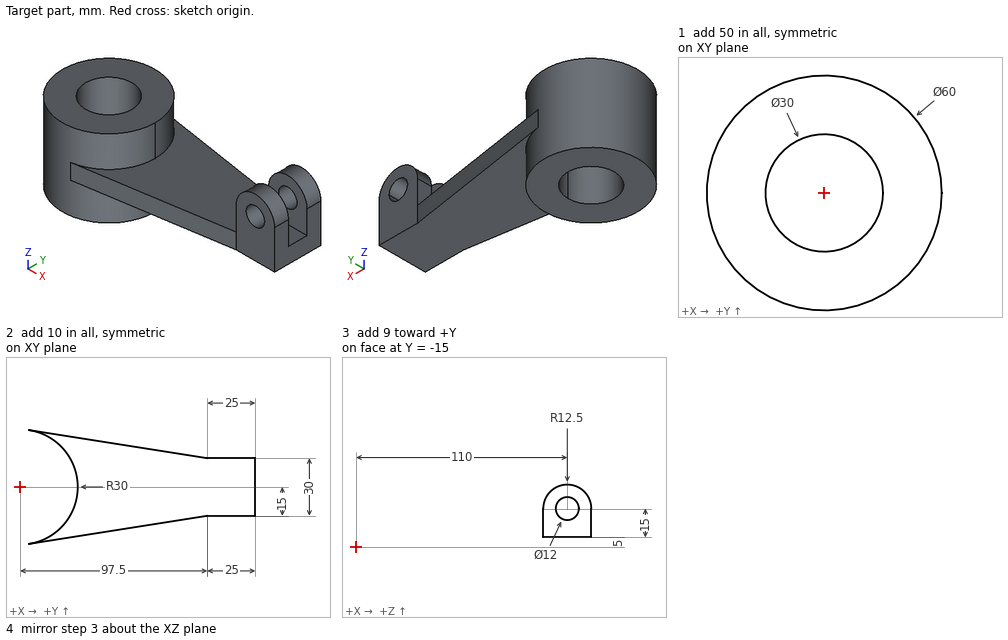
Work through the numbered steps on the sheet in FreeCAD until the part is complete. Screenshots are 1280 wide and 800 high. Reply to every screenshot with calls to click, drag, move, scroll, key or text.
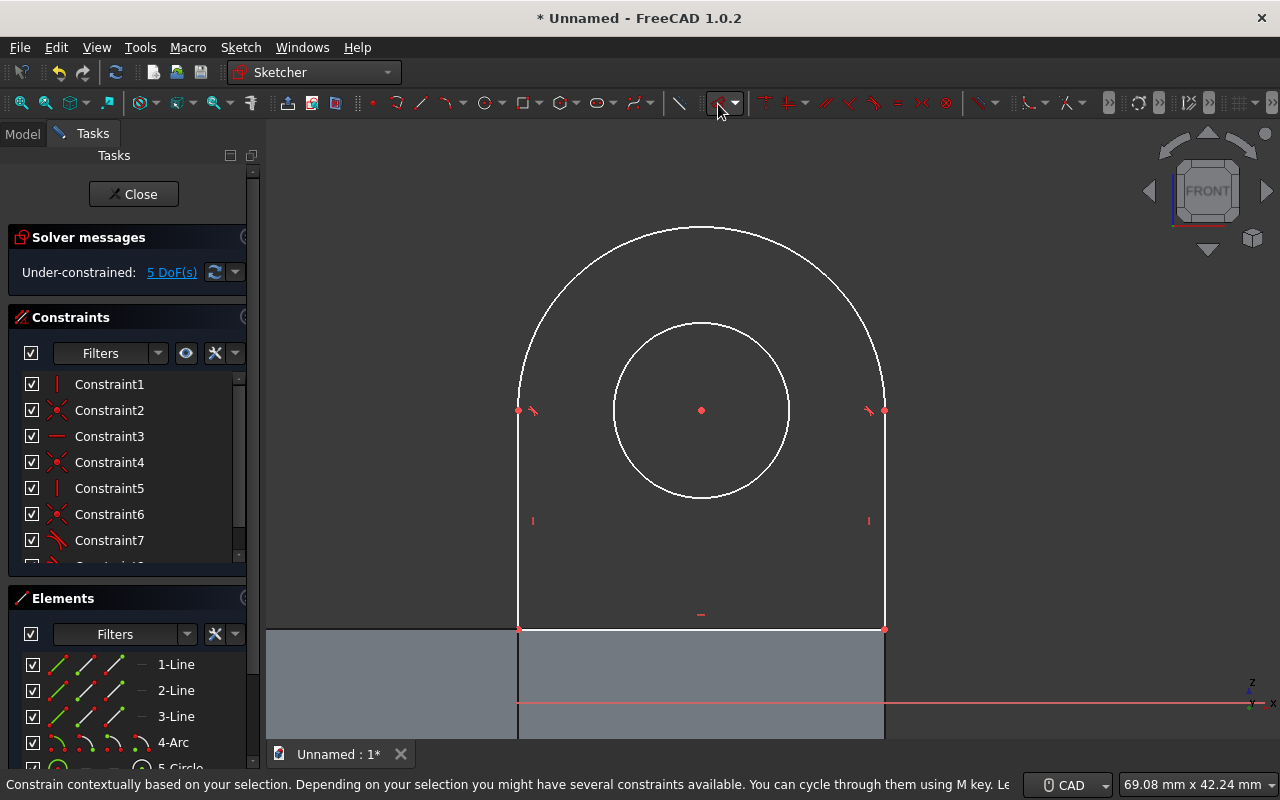
click(809, 262)
click(828, 236)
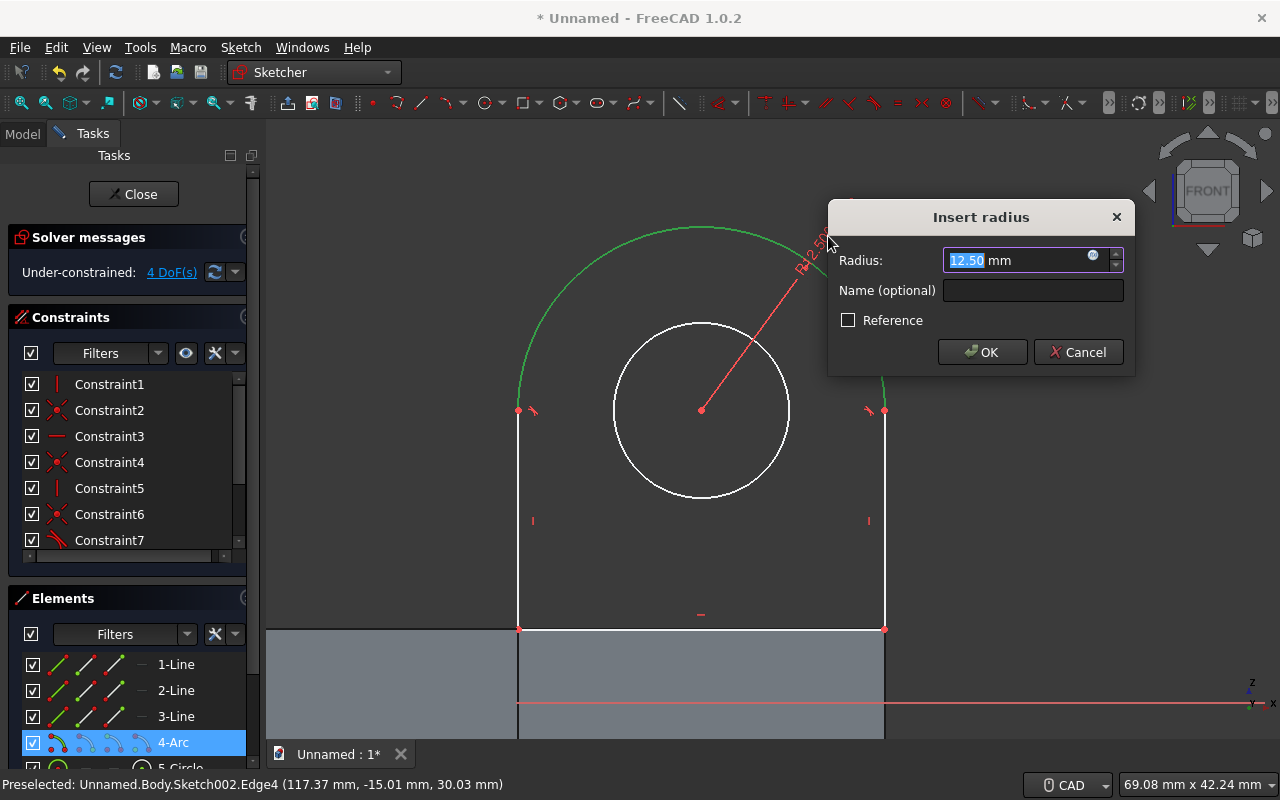
text(12.5)
key(Return)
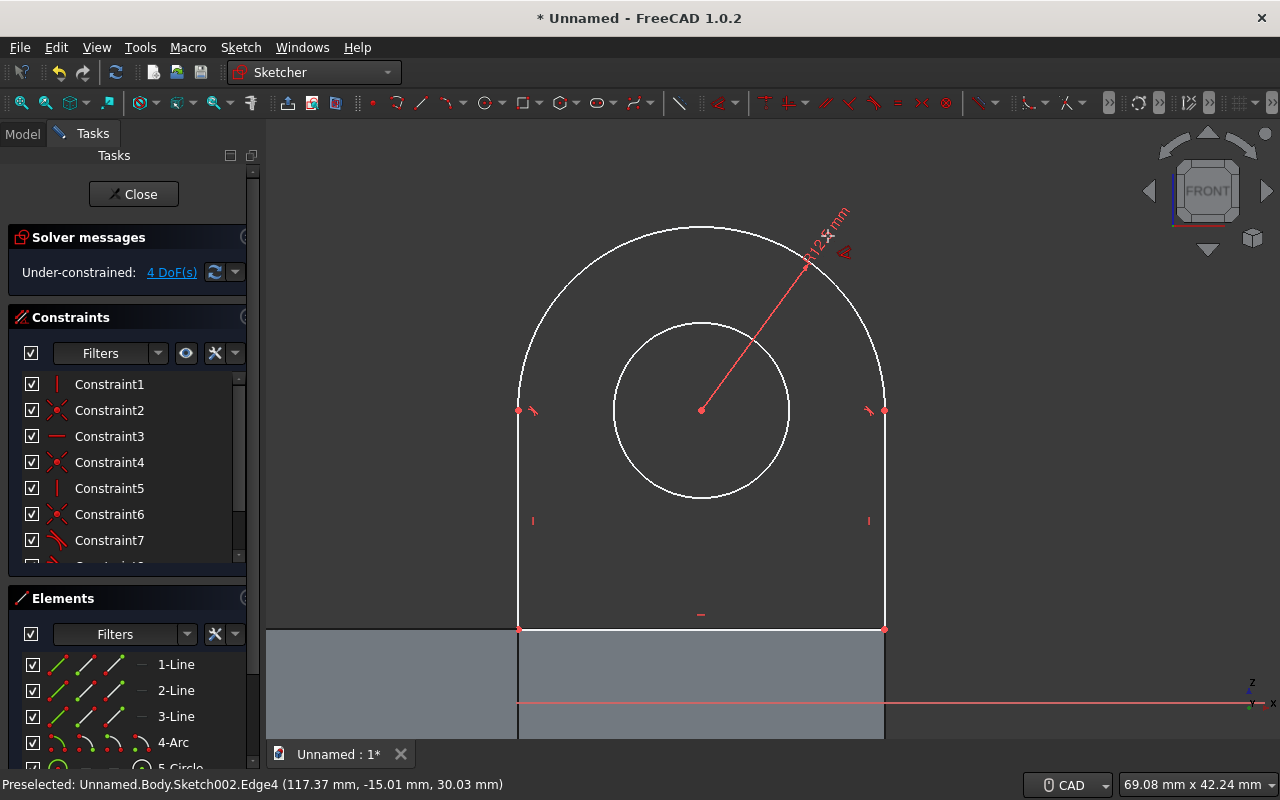
click(763, 348)
click(785, 325)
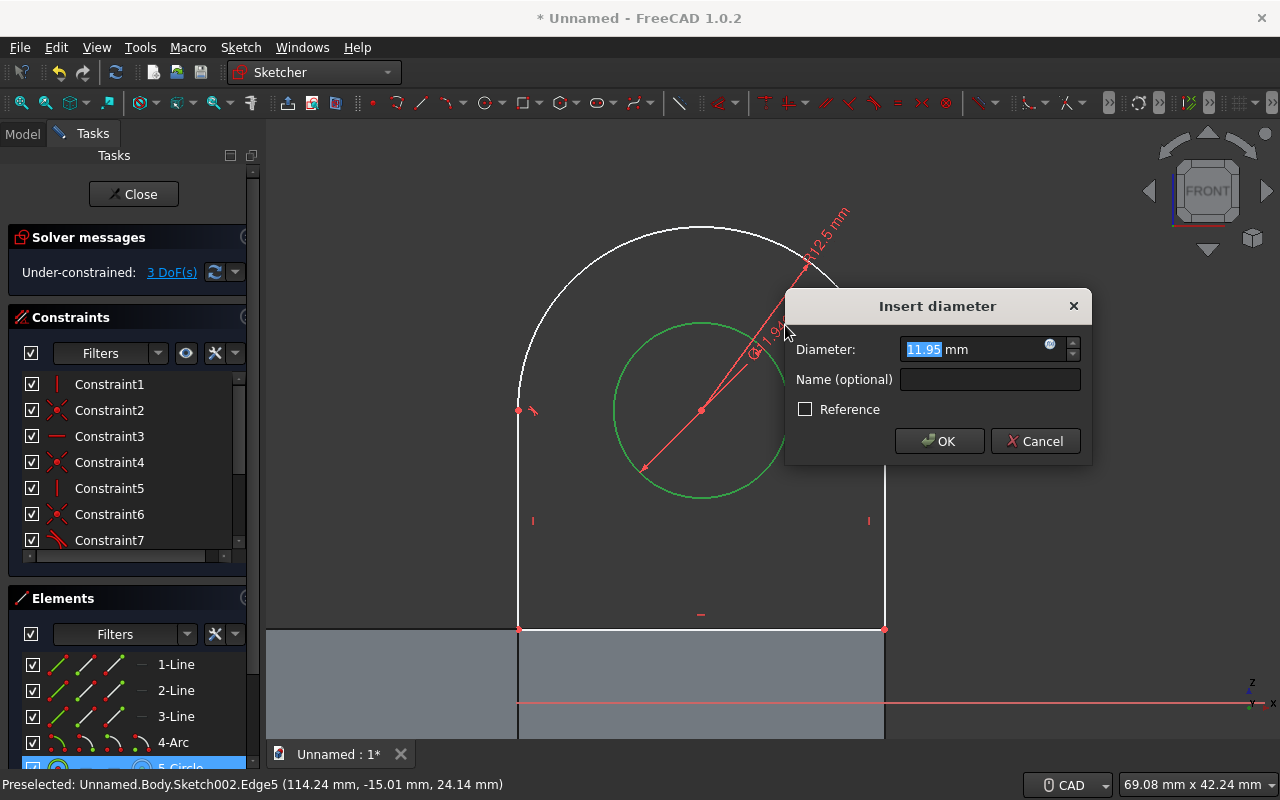
text(12)
key(Return)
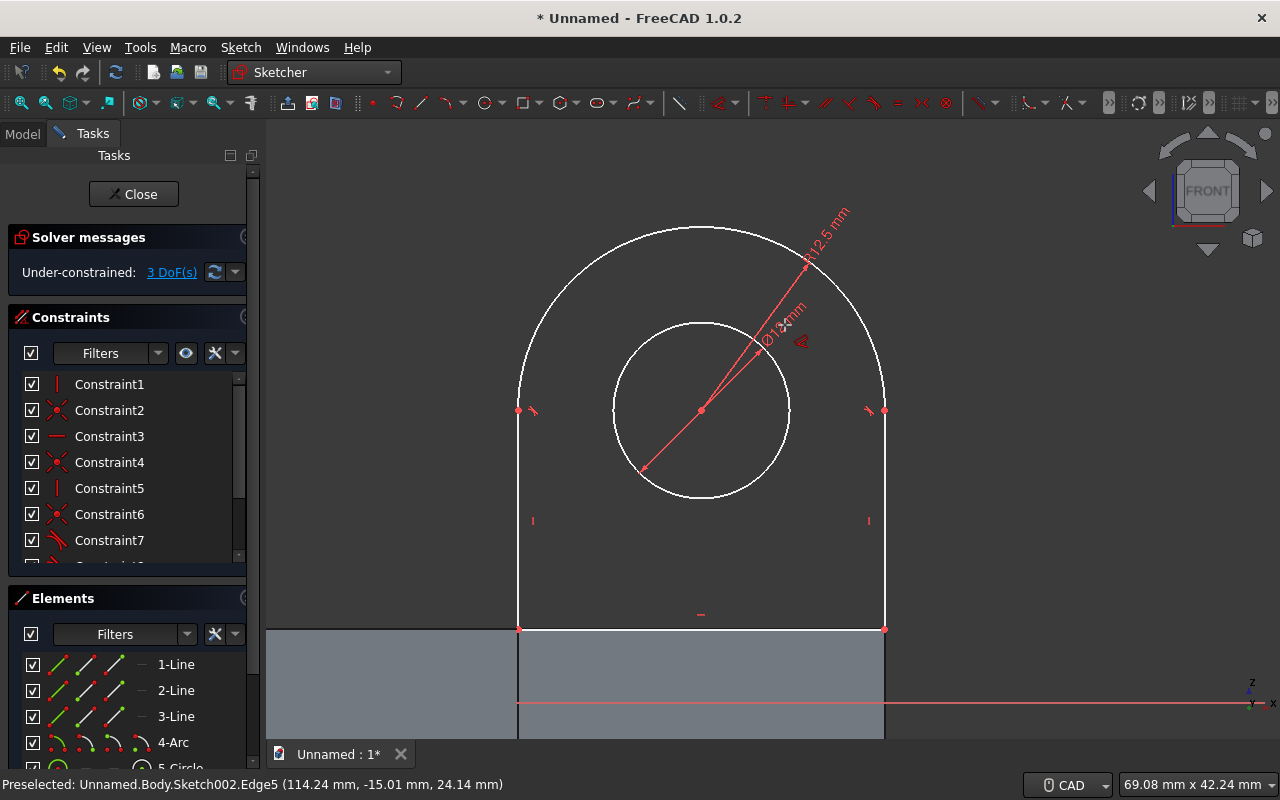
click(518, 476)
click(484, 520)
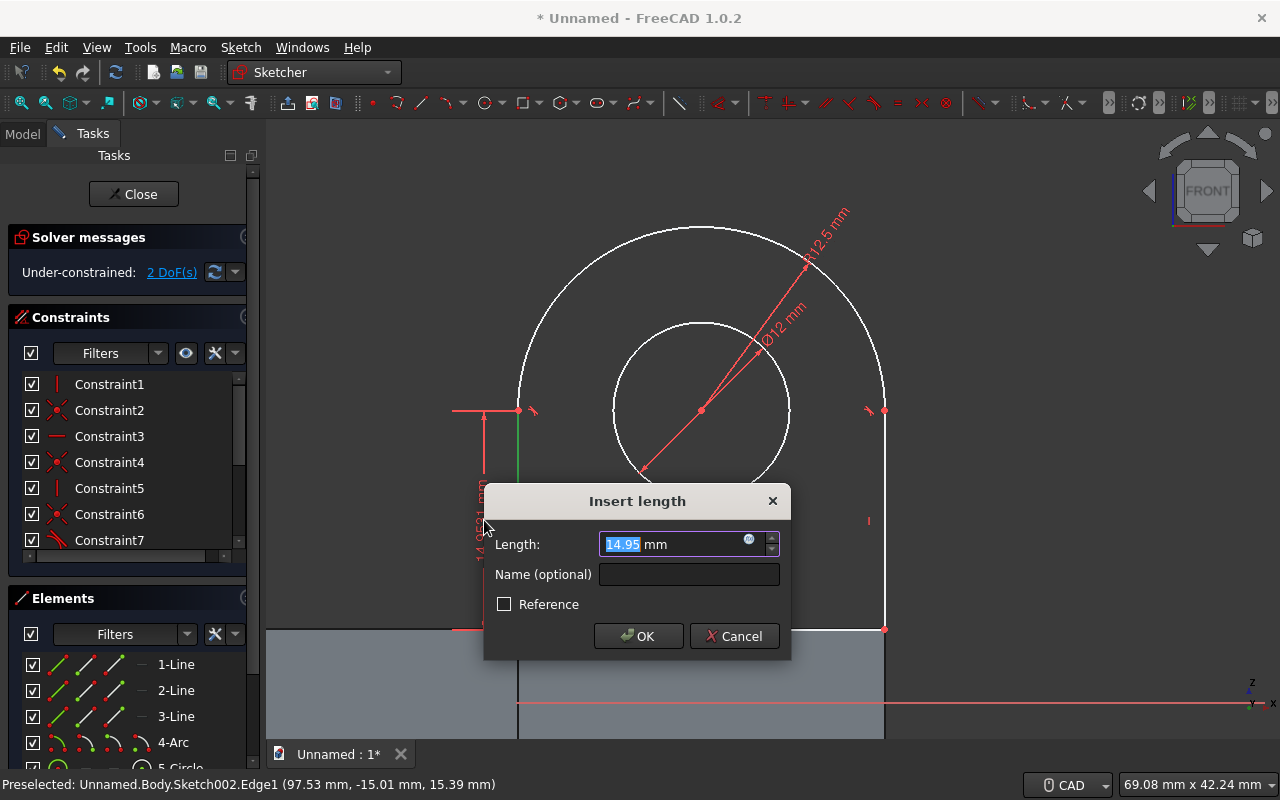
text(15)
key(Return)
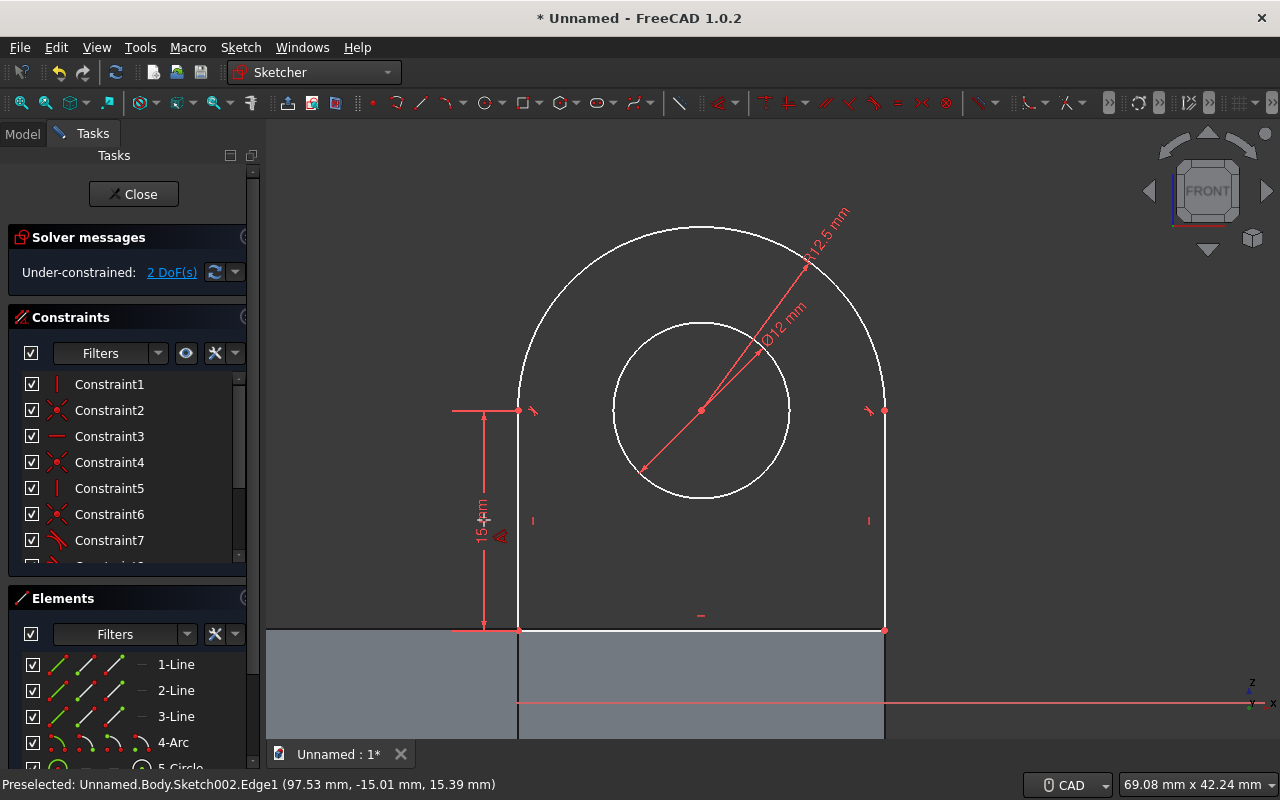
click(518, 631)
click(552, 667)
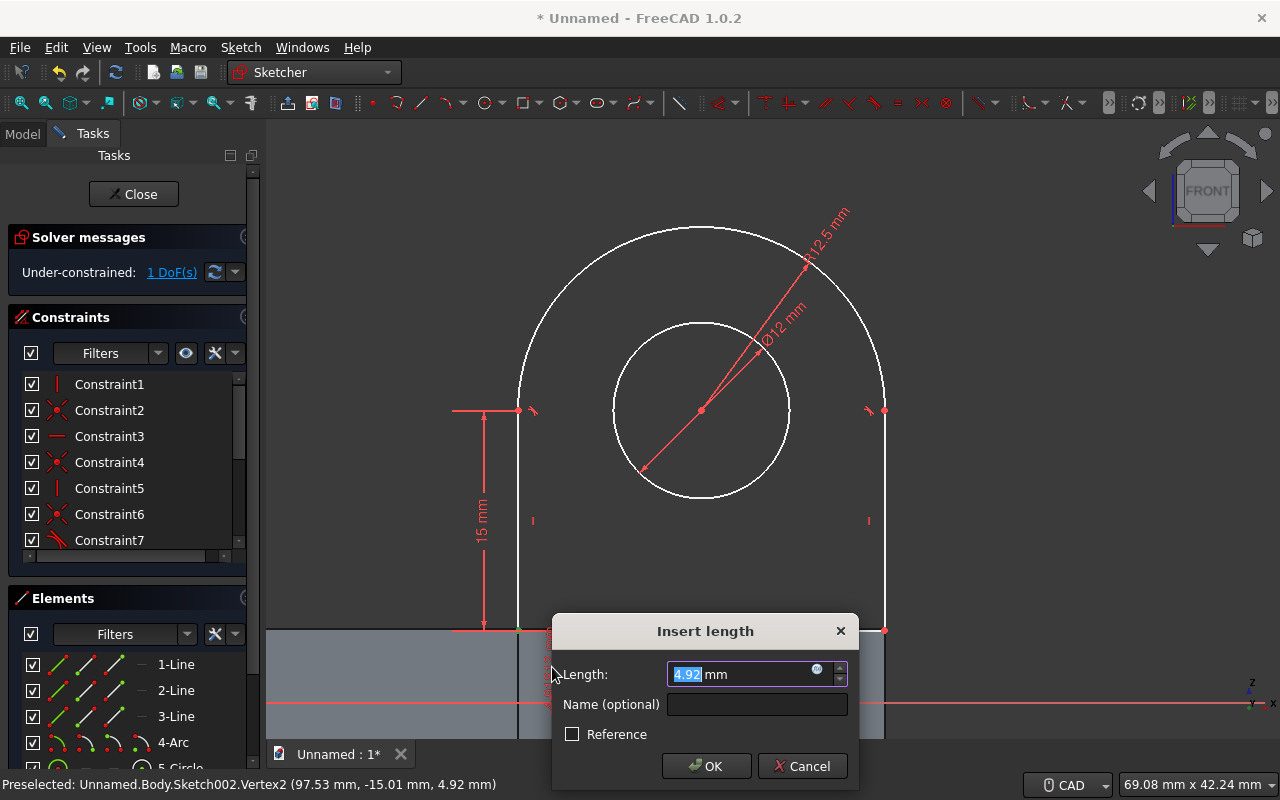
text(5)
key(Return)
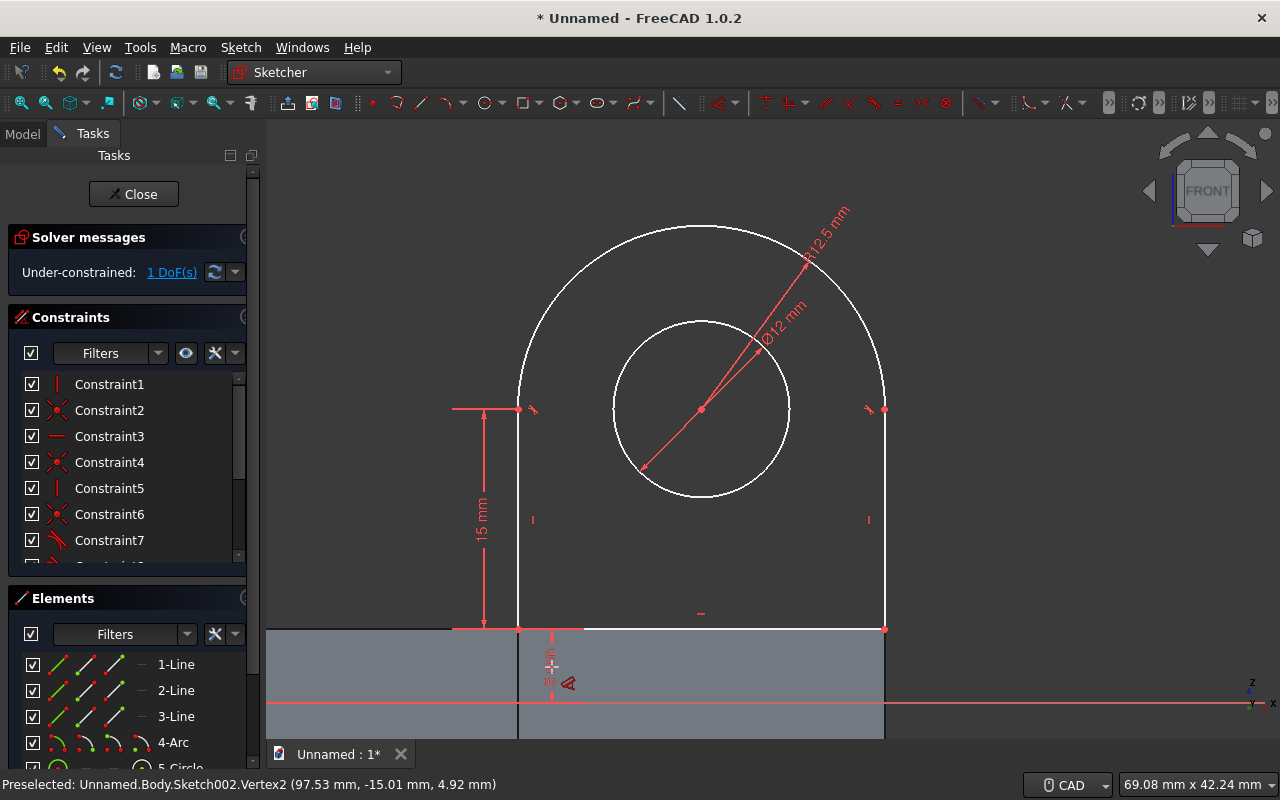
click(701, 409)
click(498, 375)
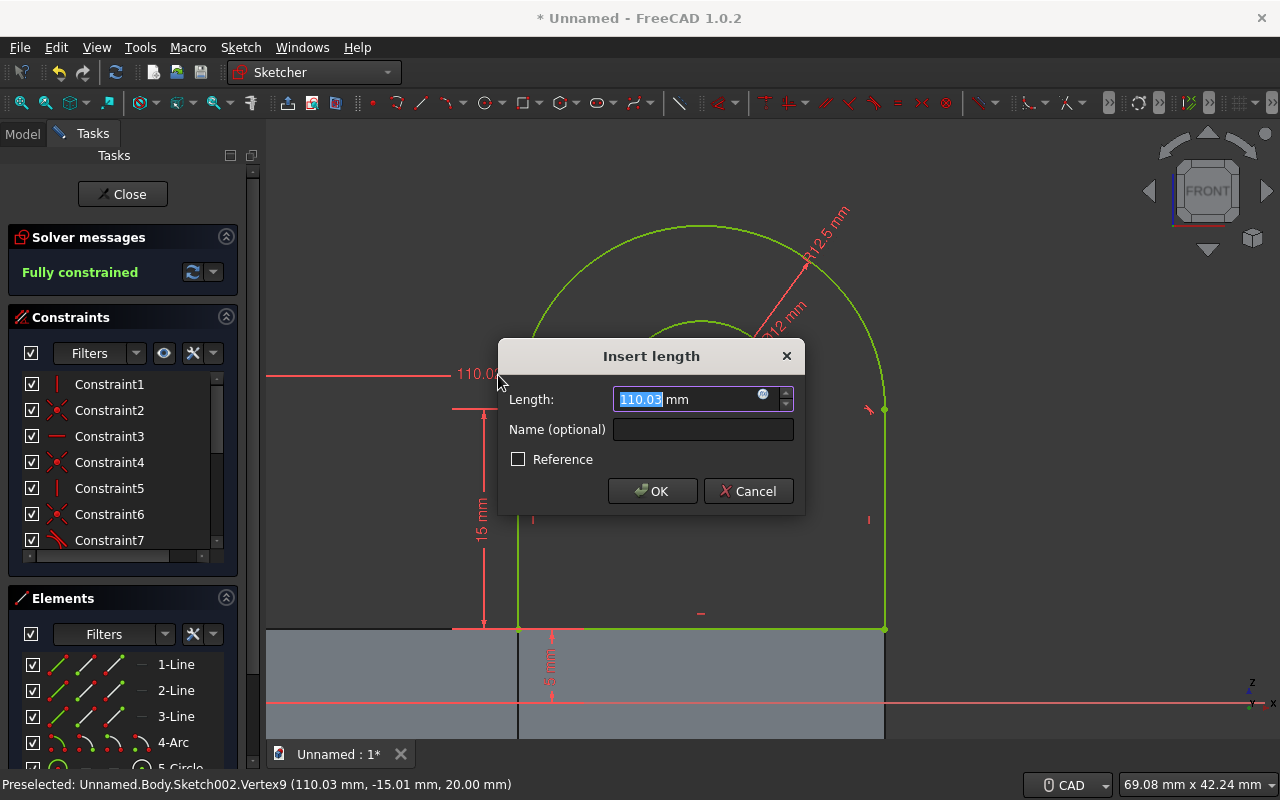
text(110)
key(Return)
key(Escape)